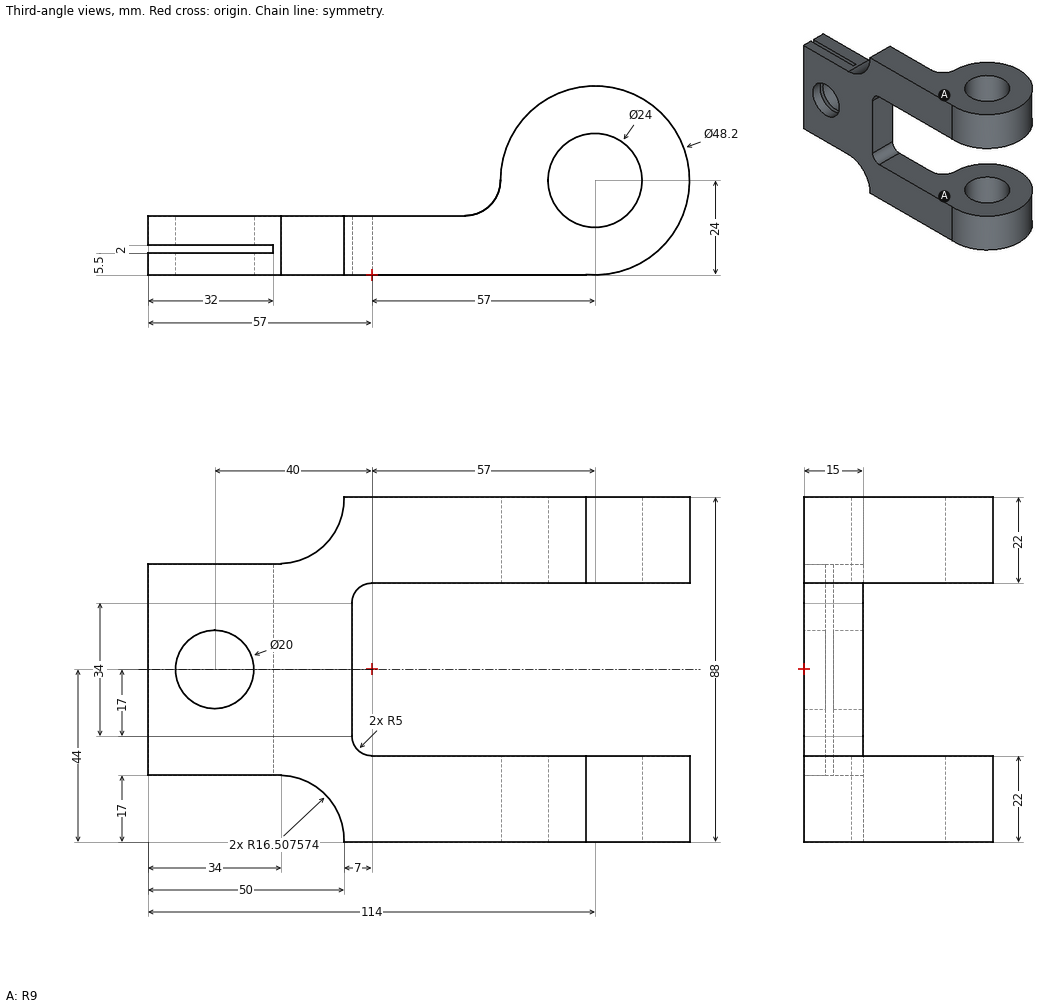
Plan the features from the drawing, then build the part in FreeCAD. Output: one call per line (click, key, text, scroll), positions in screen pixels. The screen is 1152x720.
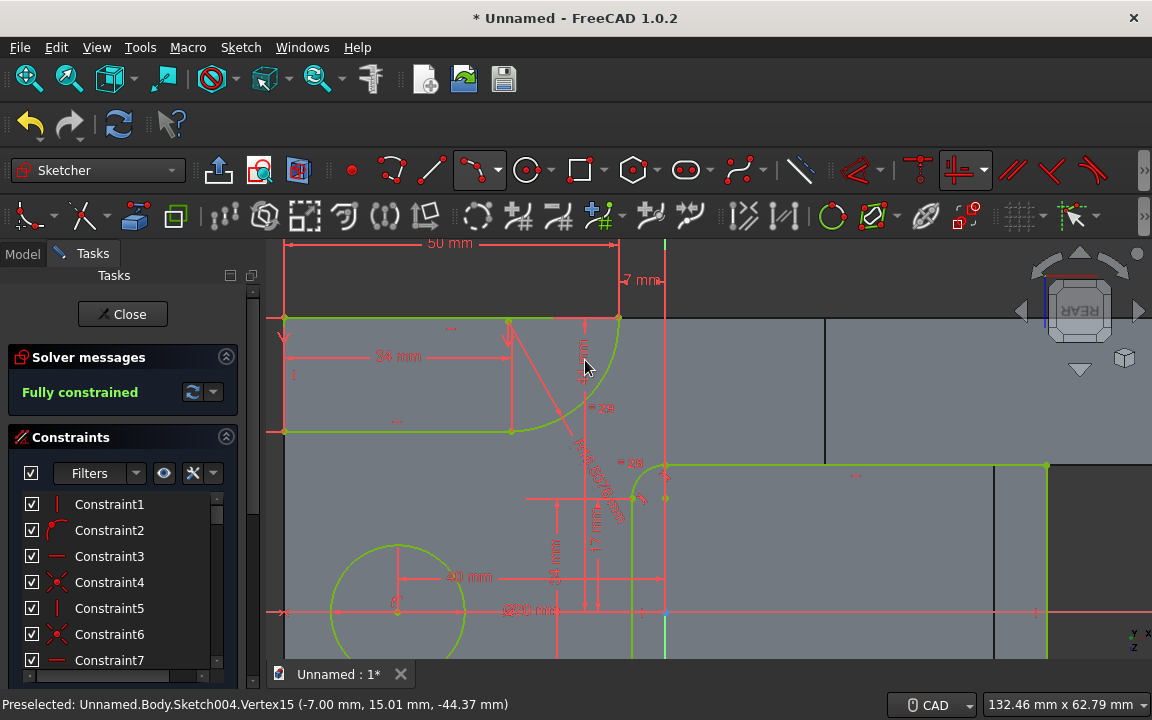
click(123, 314)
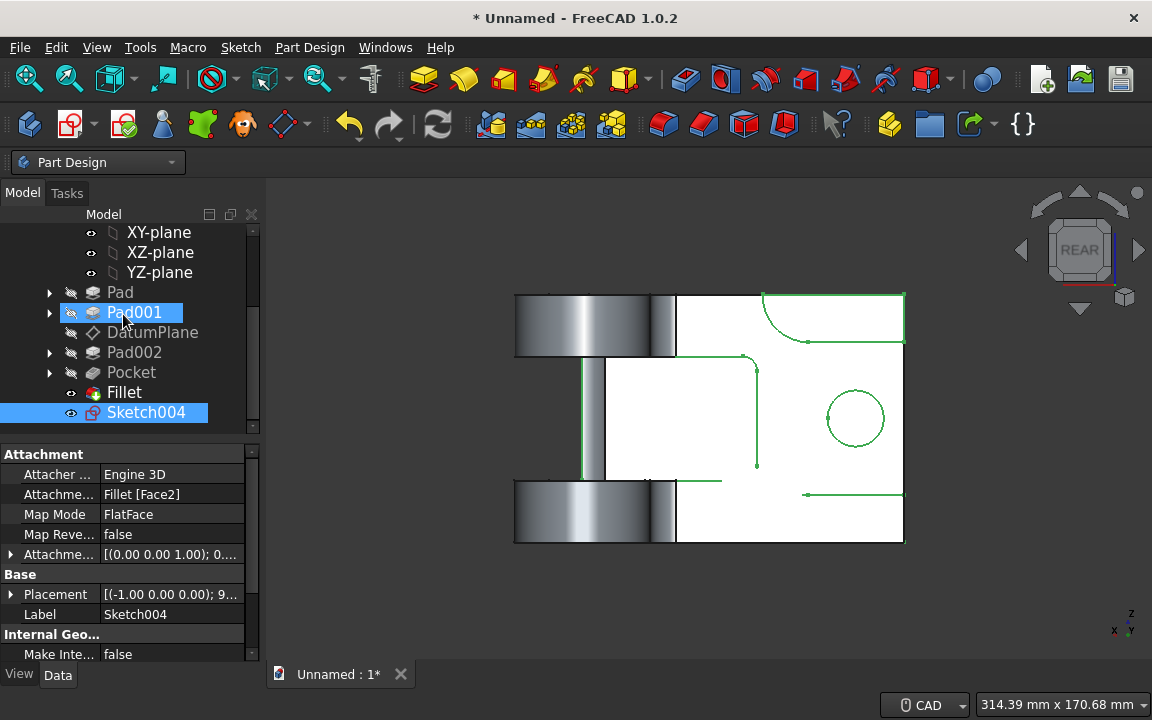
click(686, 80)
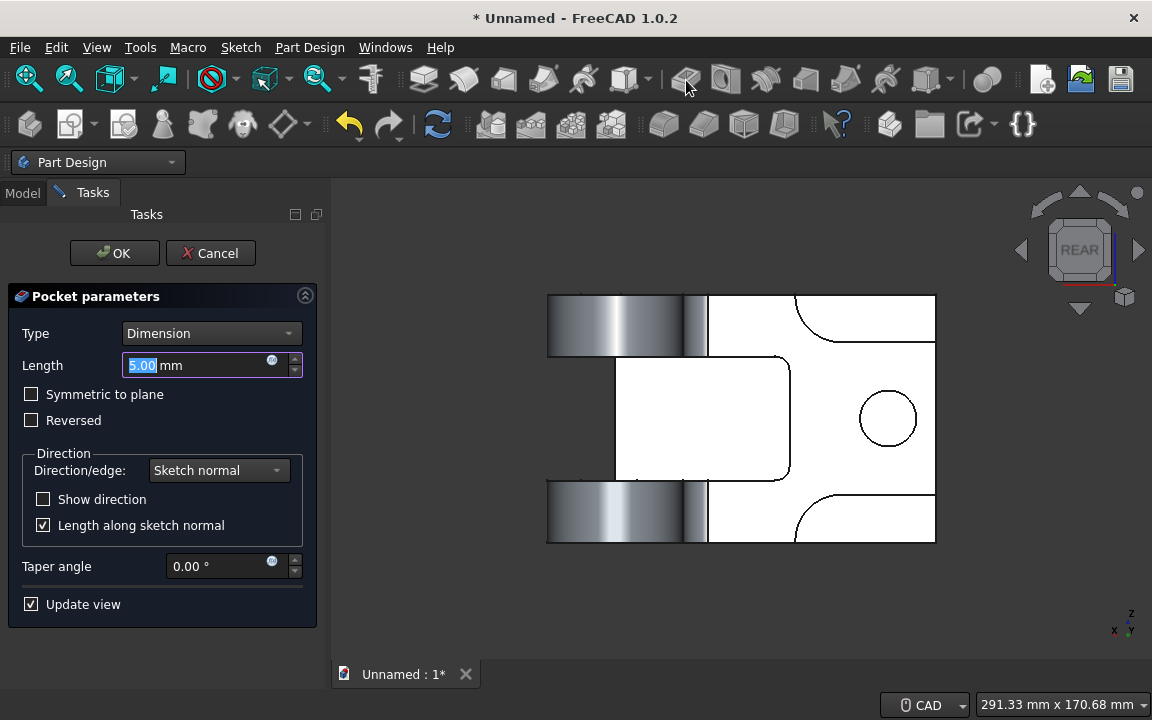
click(212, 334)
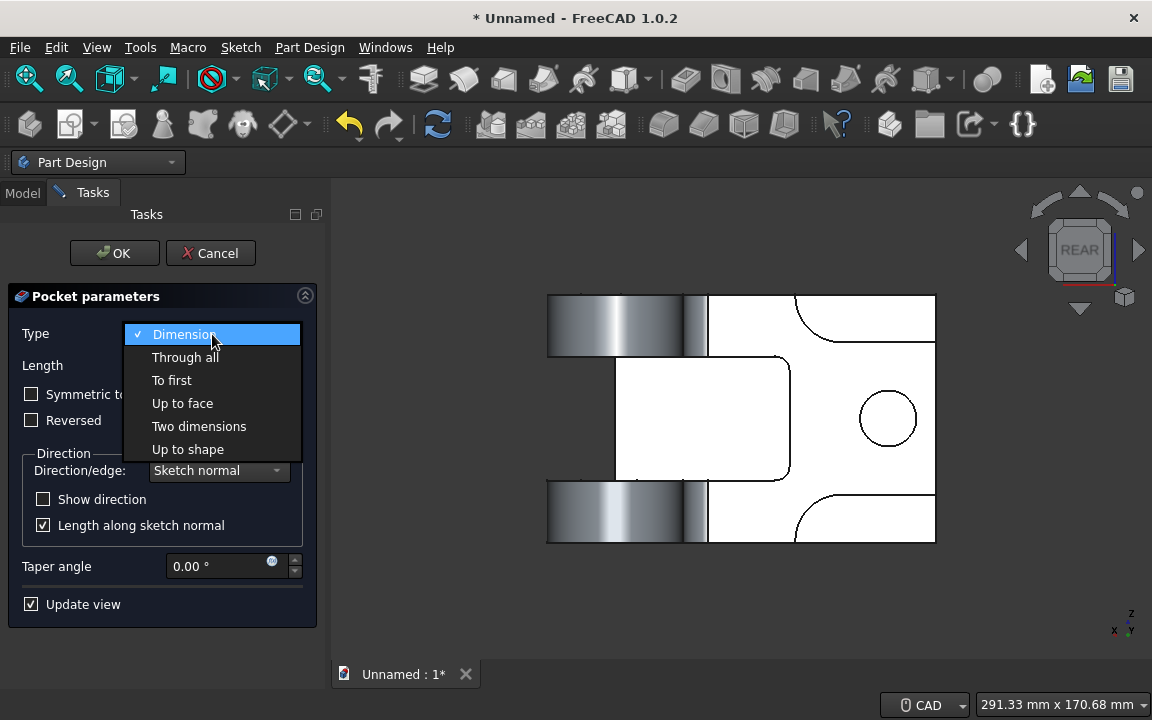
click(212, 358)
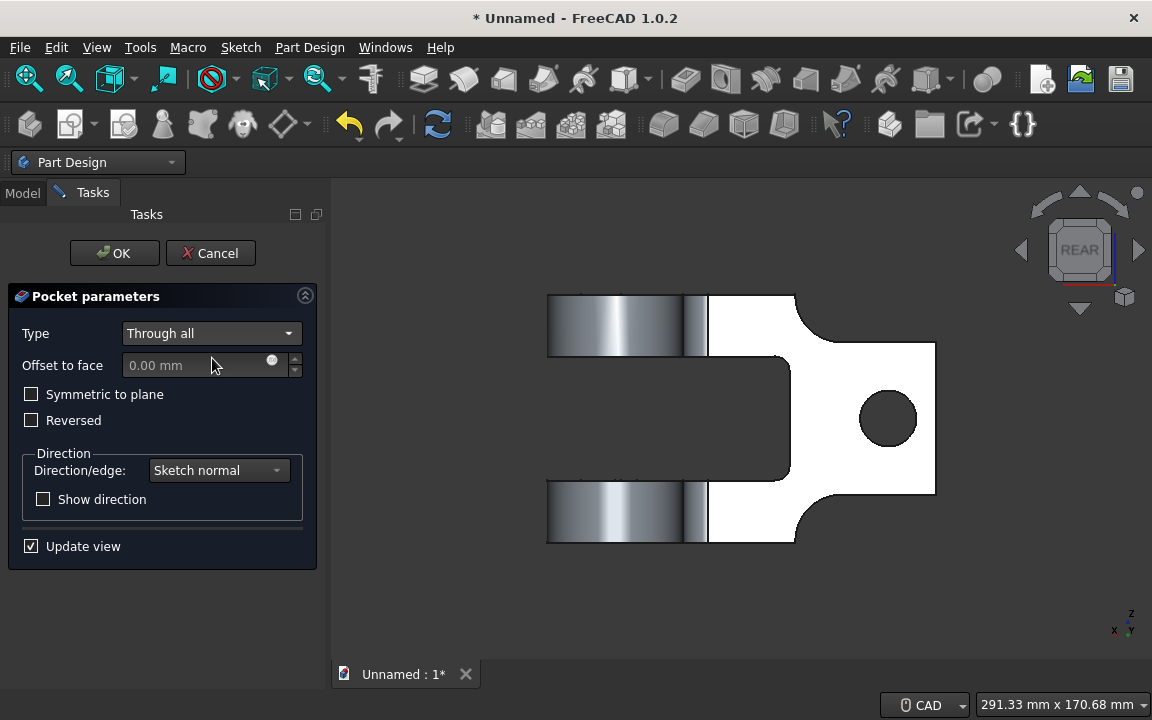
click(115, 253)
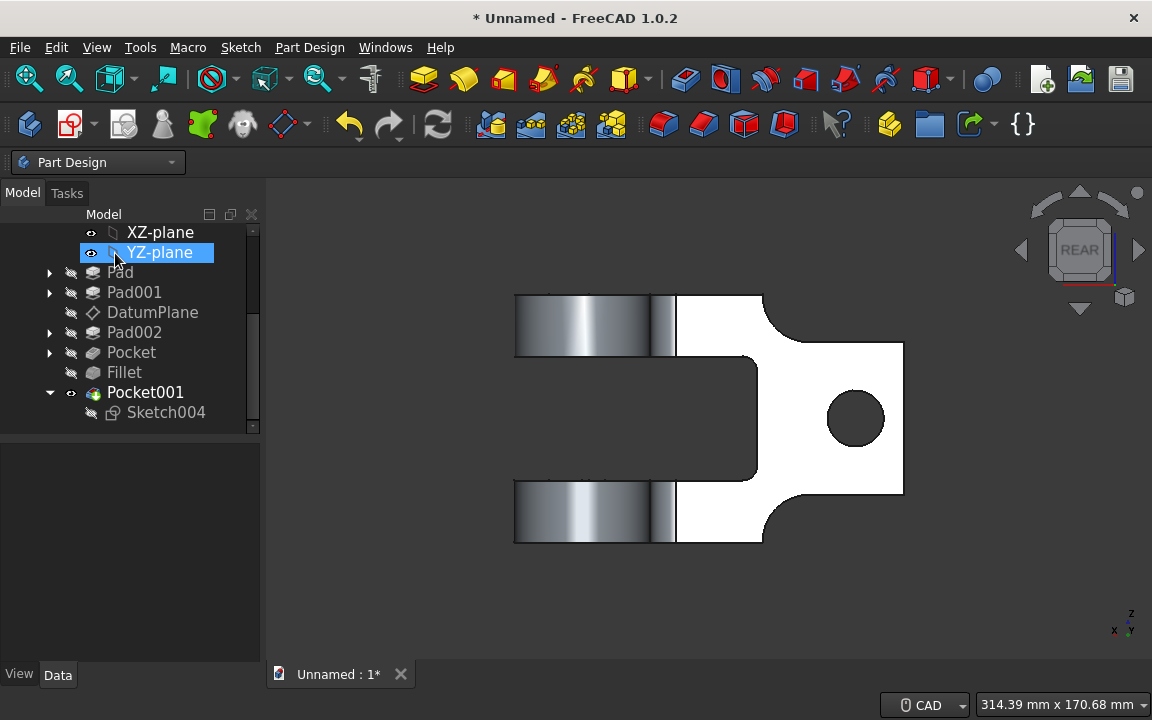
key(5)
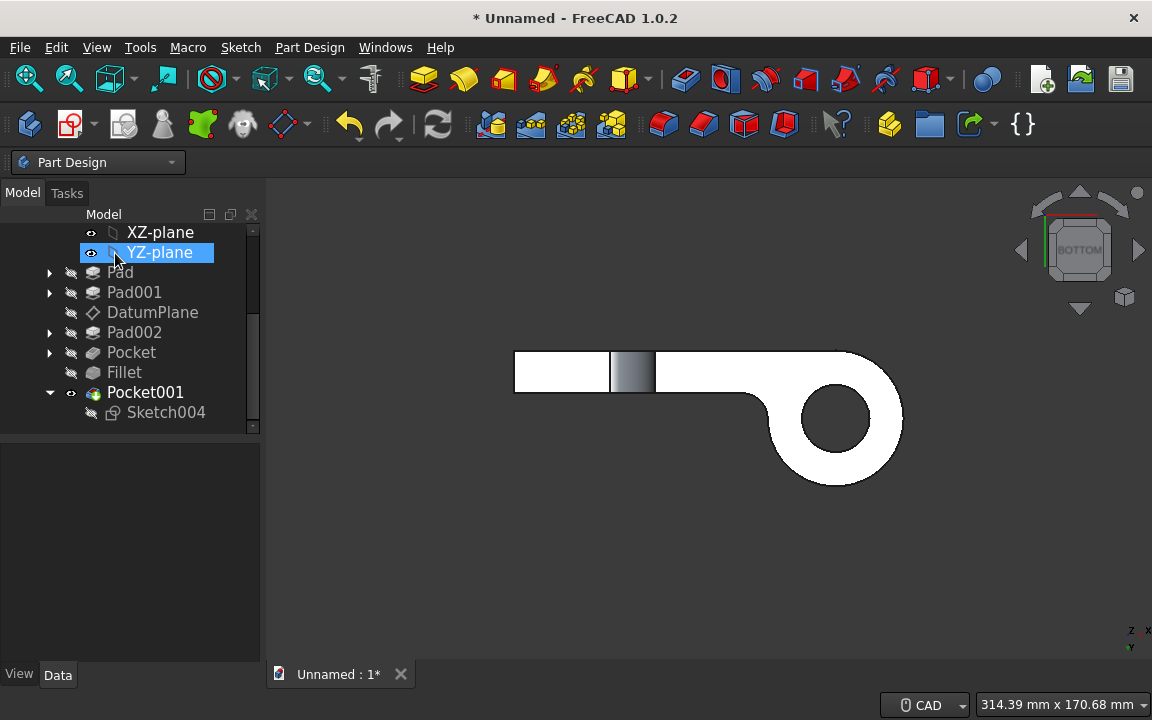
key(v)
key(f)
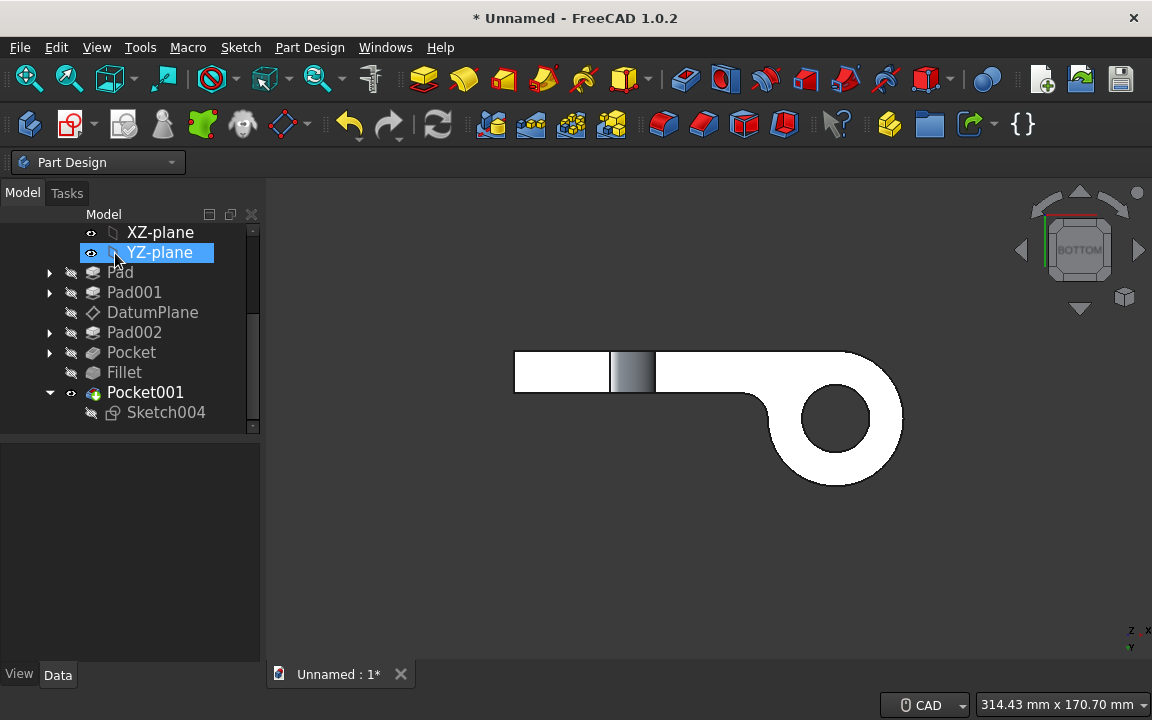
click(576, 371)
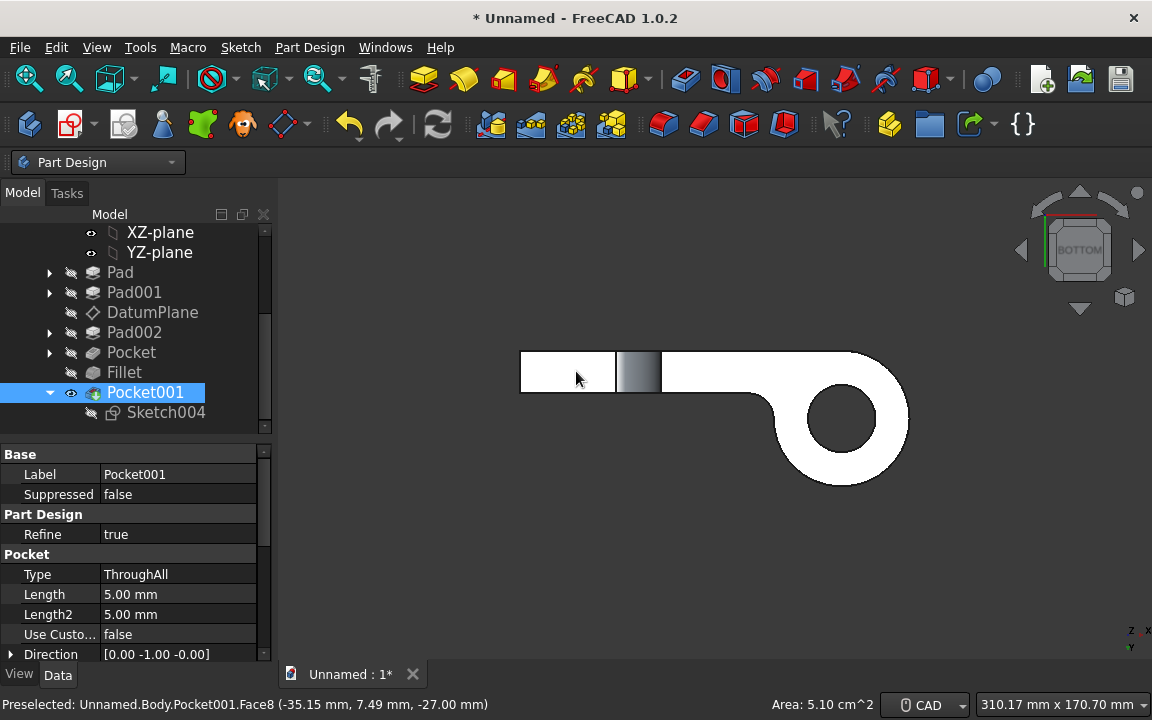
click(70, 124)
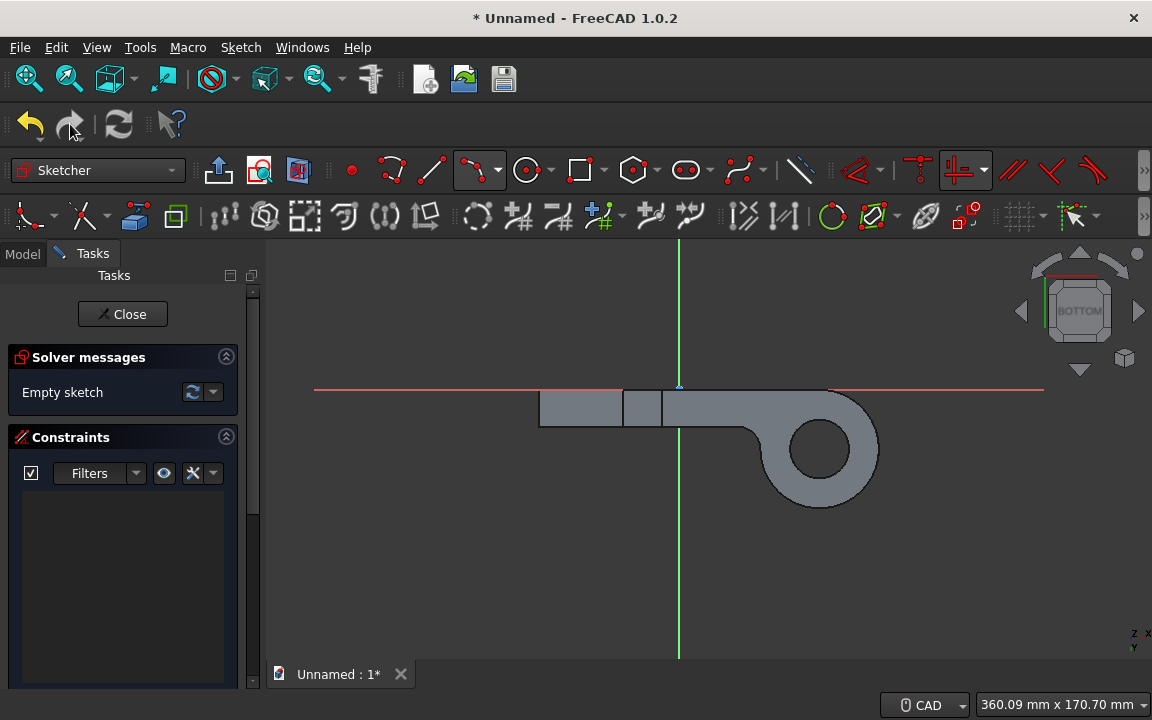
key(q)
key(s)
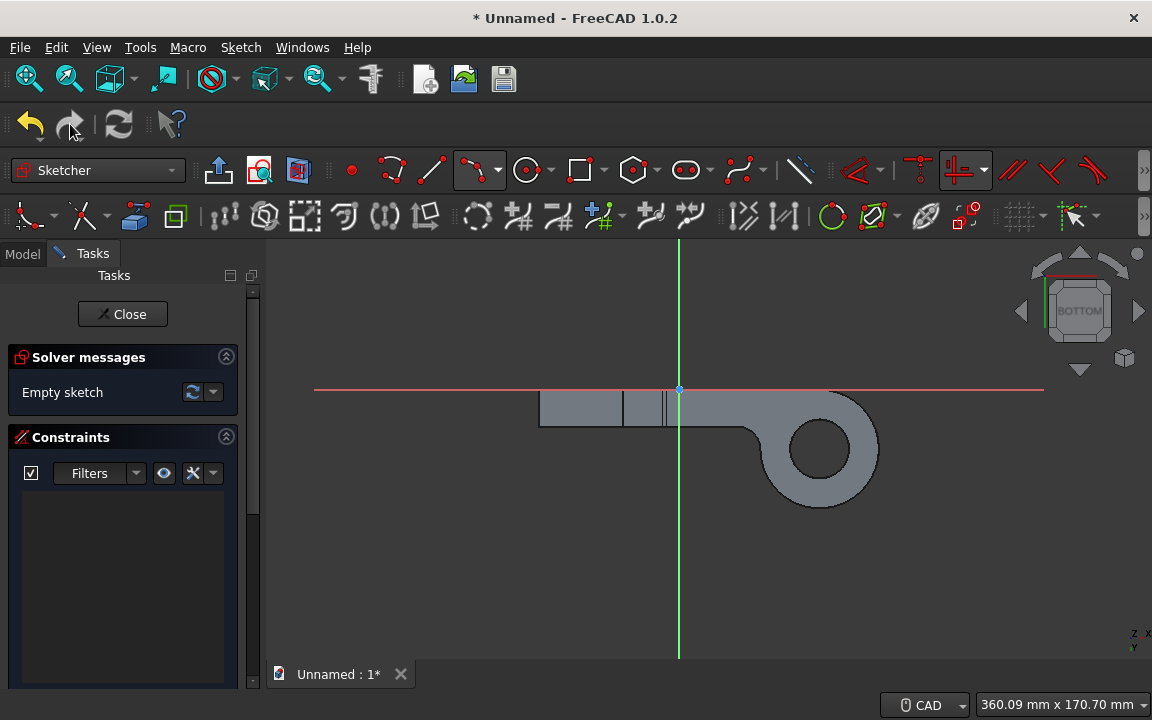
scroll(596, 378, up, 6)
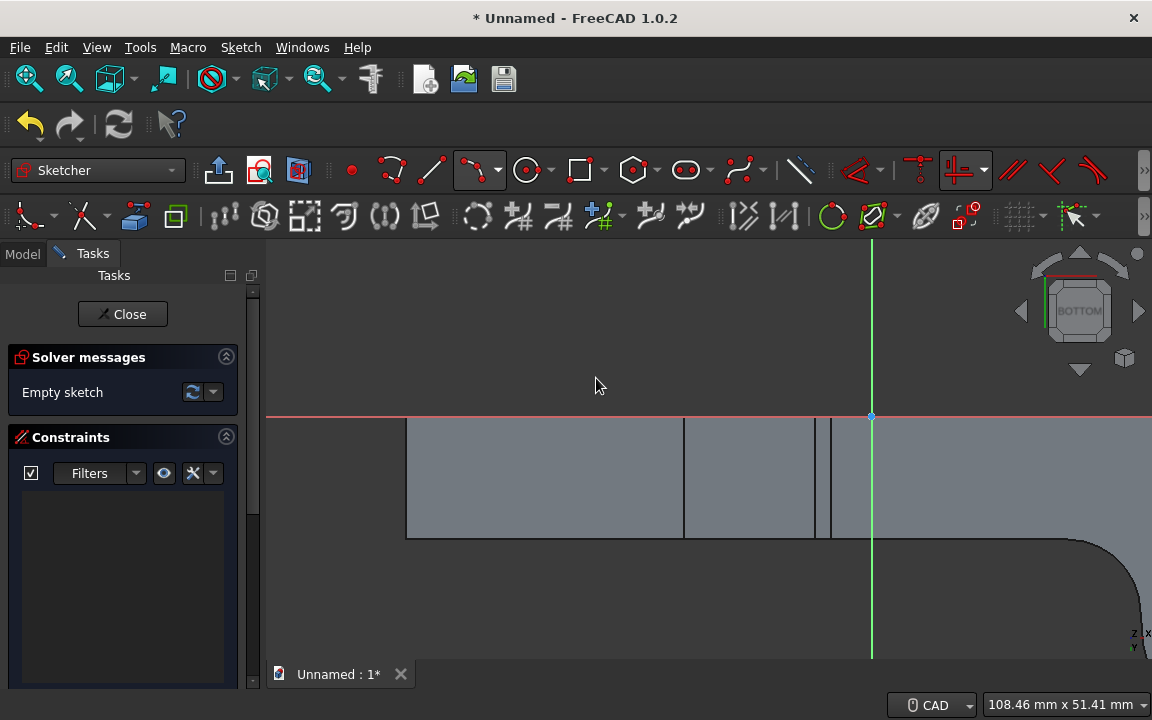
click(580, 170)